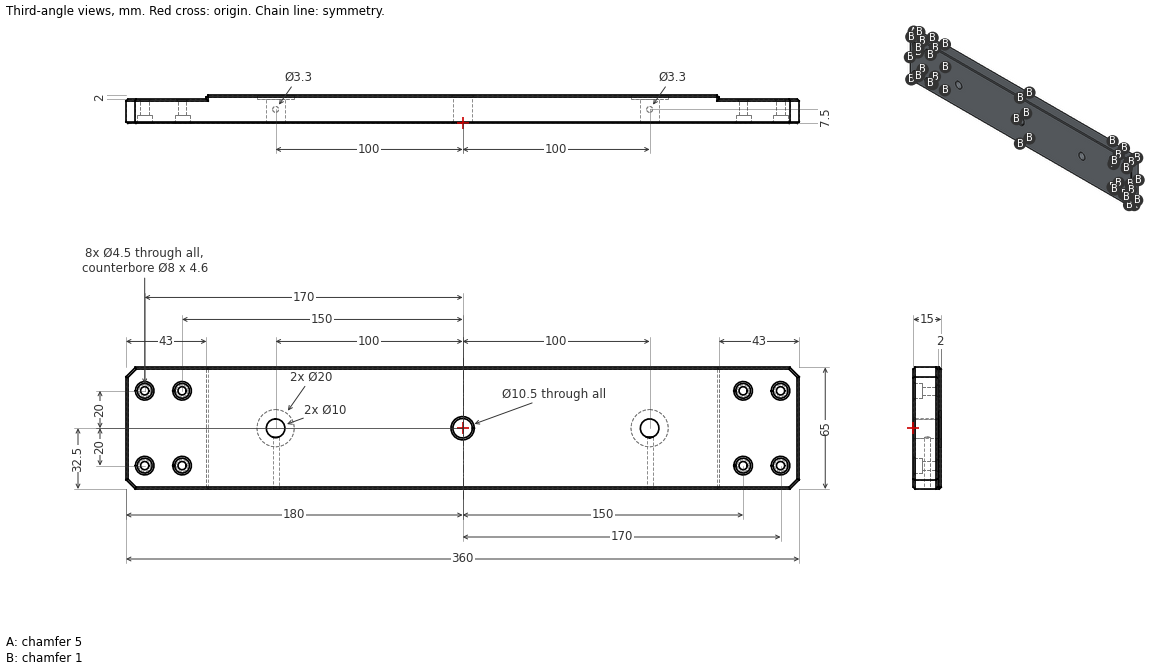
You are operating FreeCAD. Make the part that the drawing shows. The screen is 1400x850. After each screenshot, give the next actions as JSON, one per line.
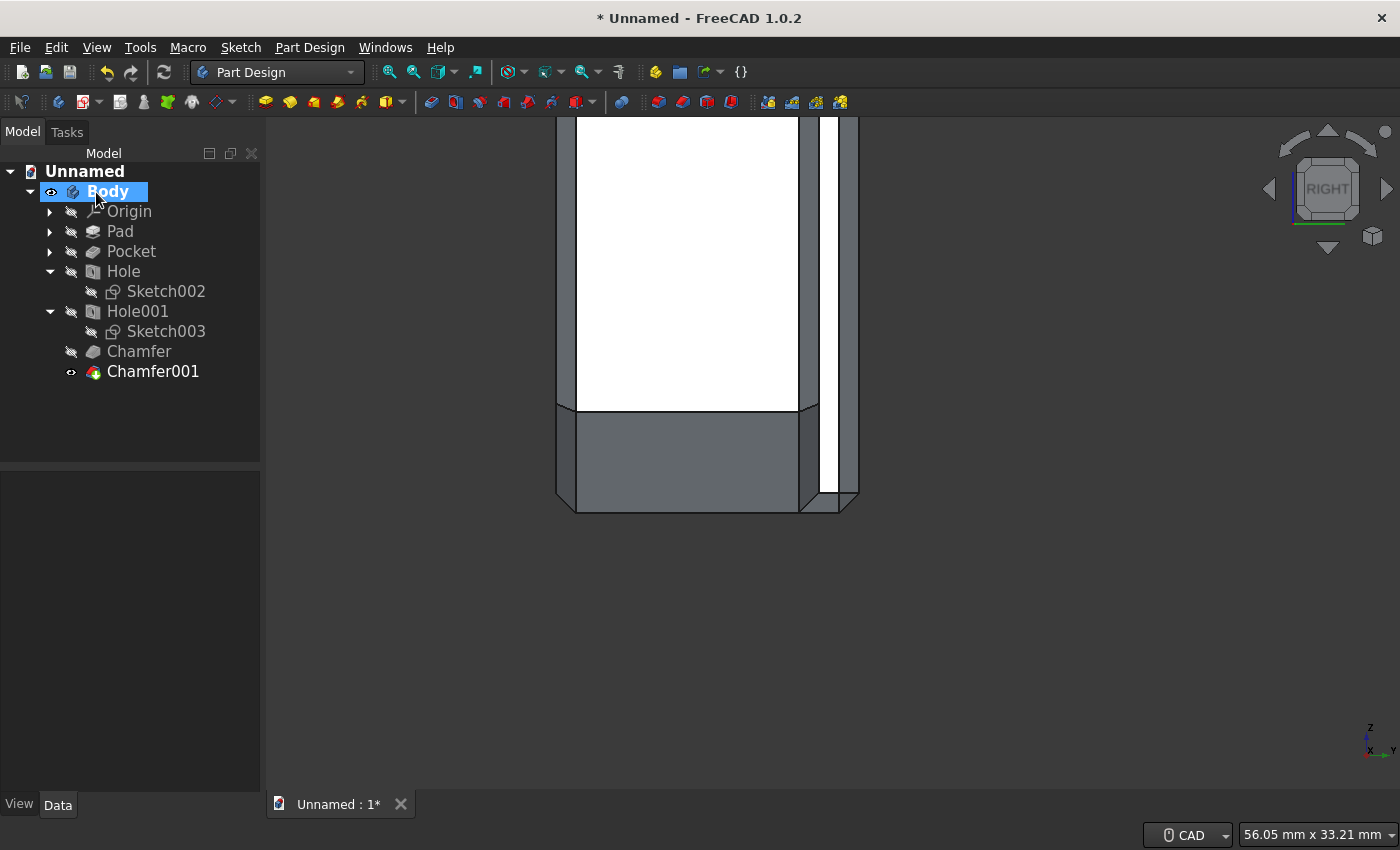
{"action": "left_click", "coordinate": [390, 72]}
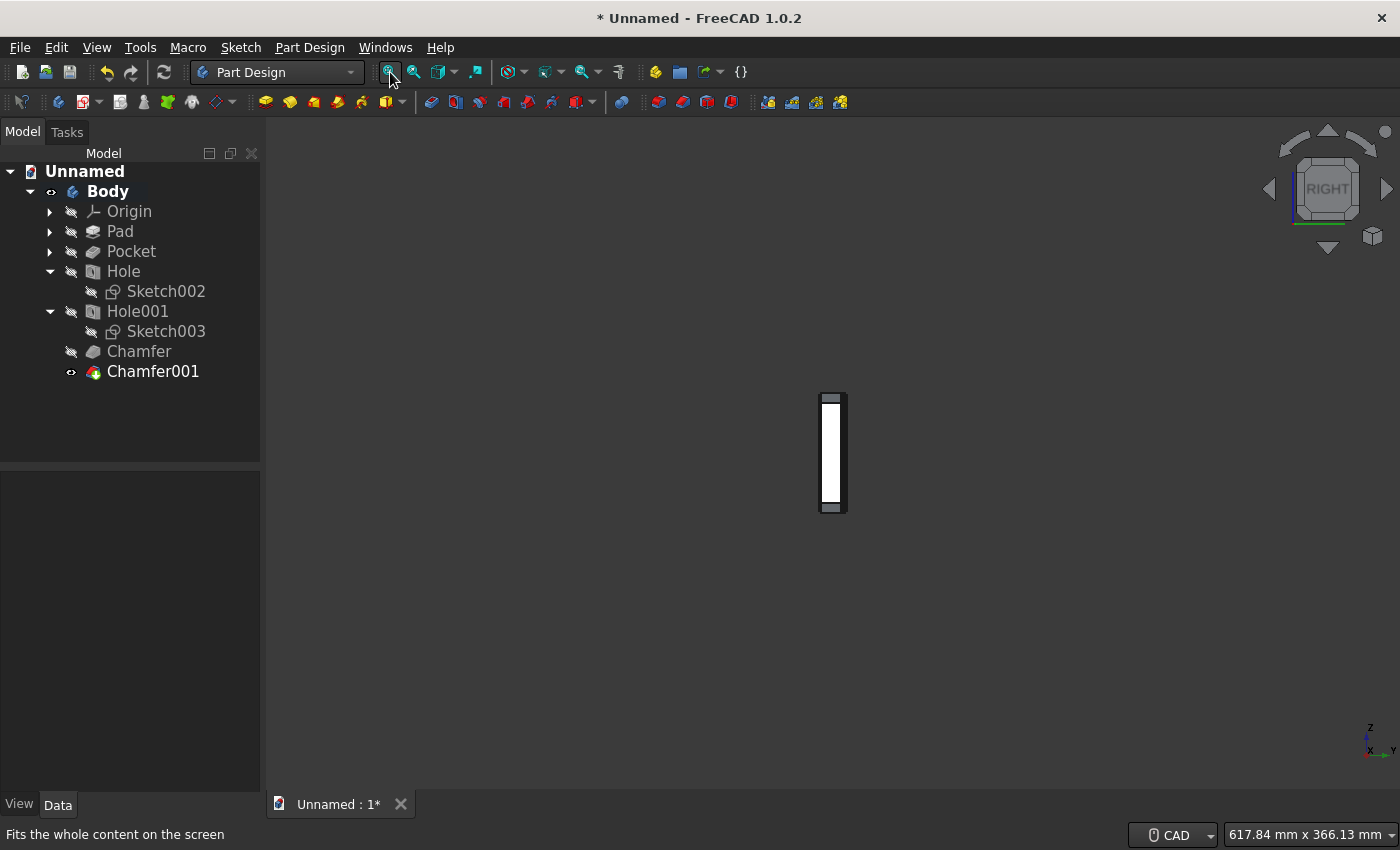
{"action": "key", "text": "4"}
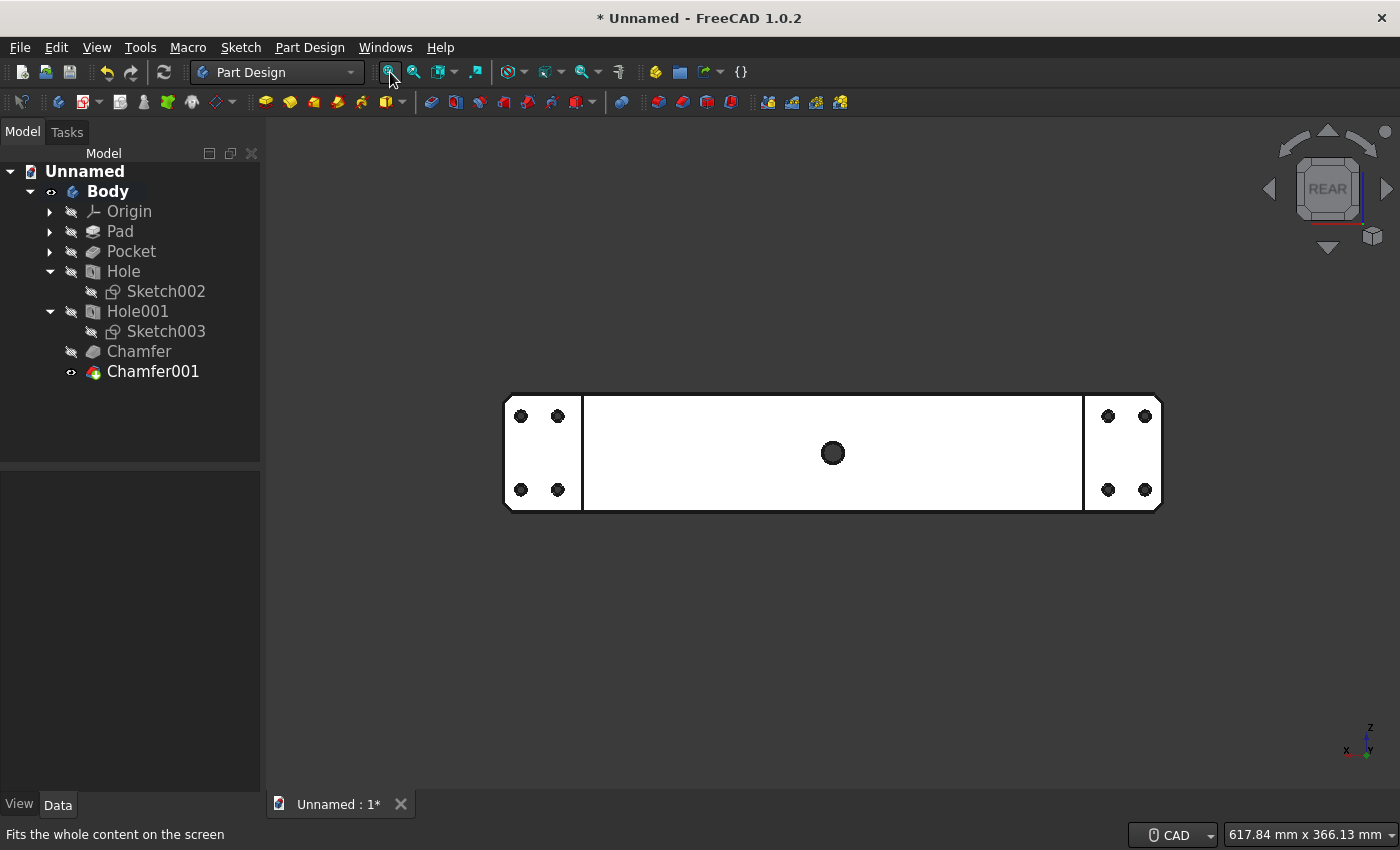
{"action": "left_click", "coordinate": [690, 452]}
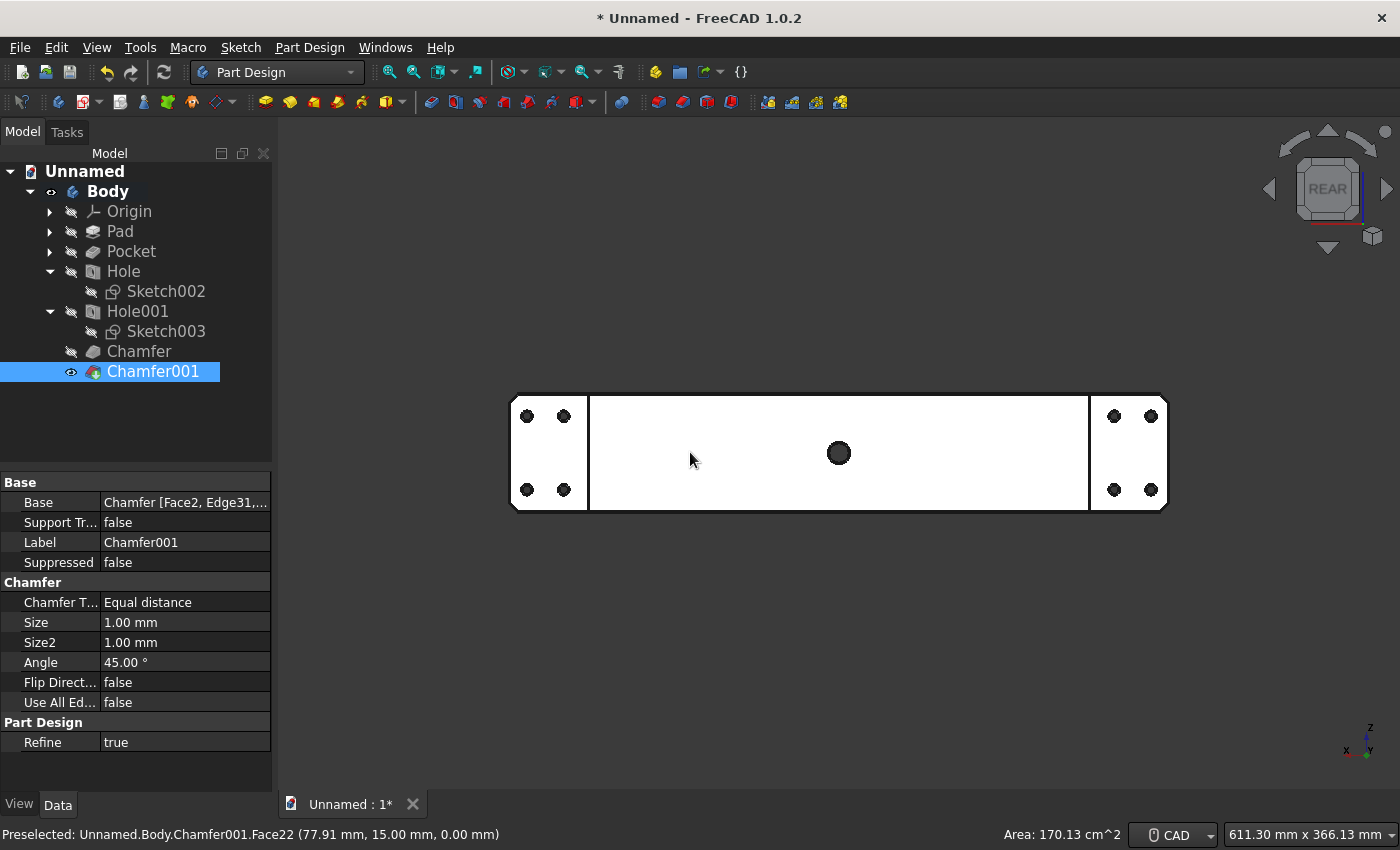
{"action": "left_click", "coordinate": [84, 102]}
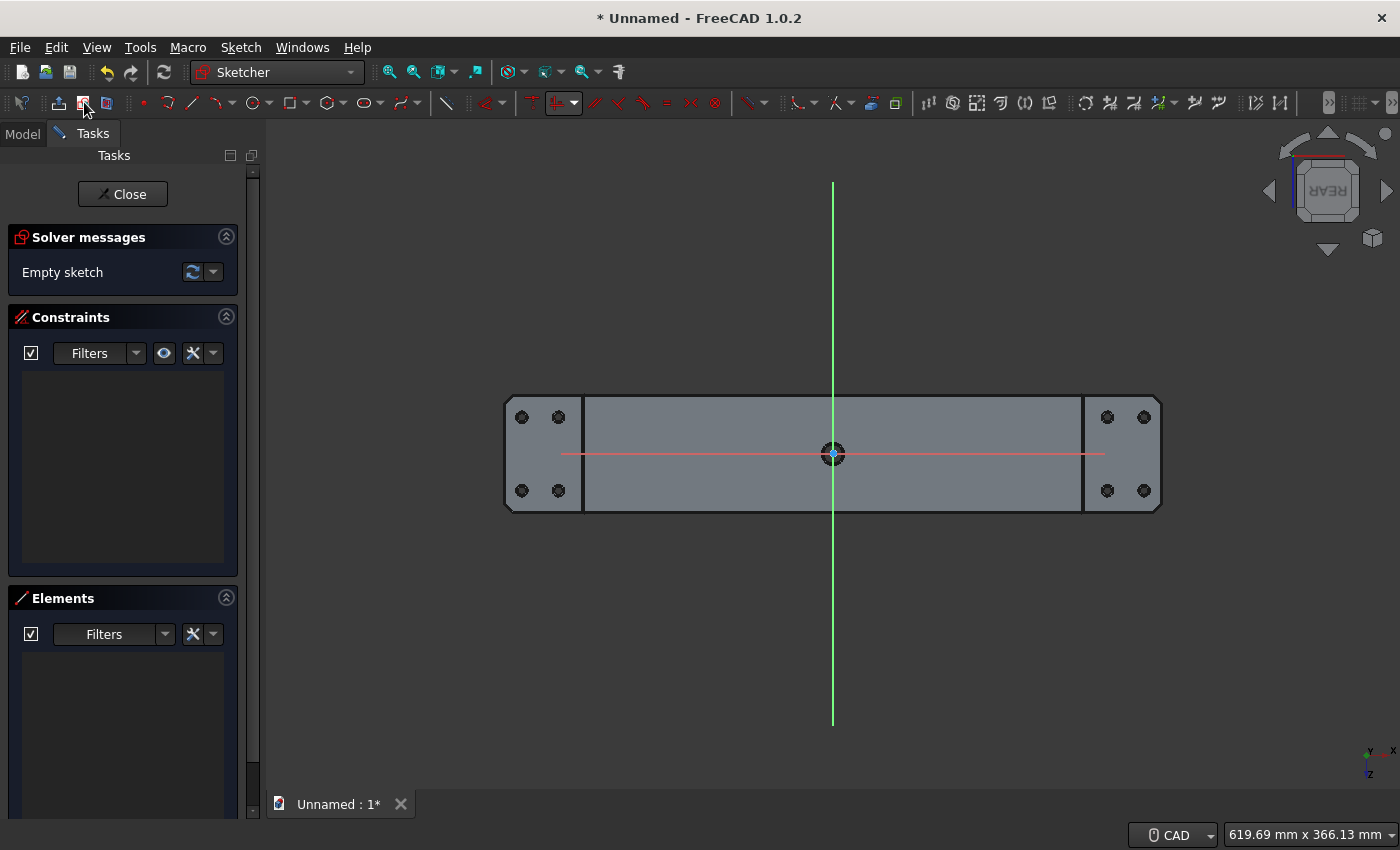
{"action": "scroll", "coordinate": [916, 454], "scroll_direction": "up", "scroll_amount": 3}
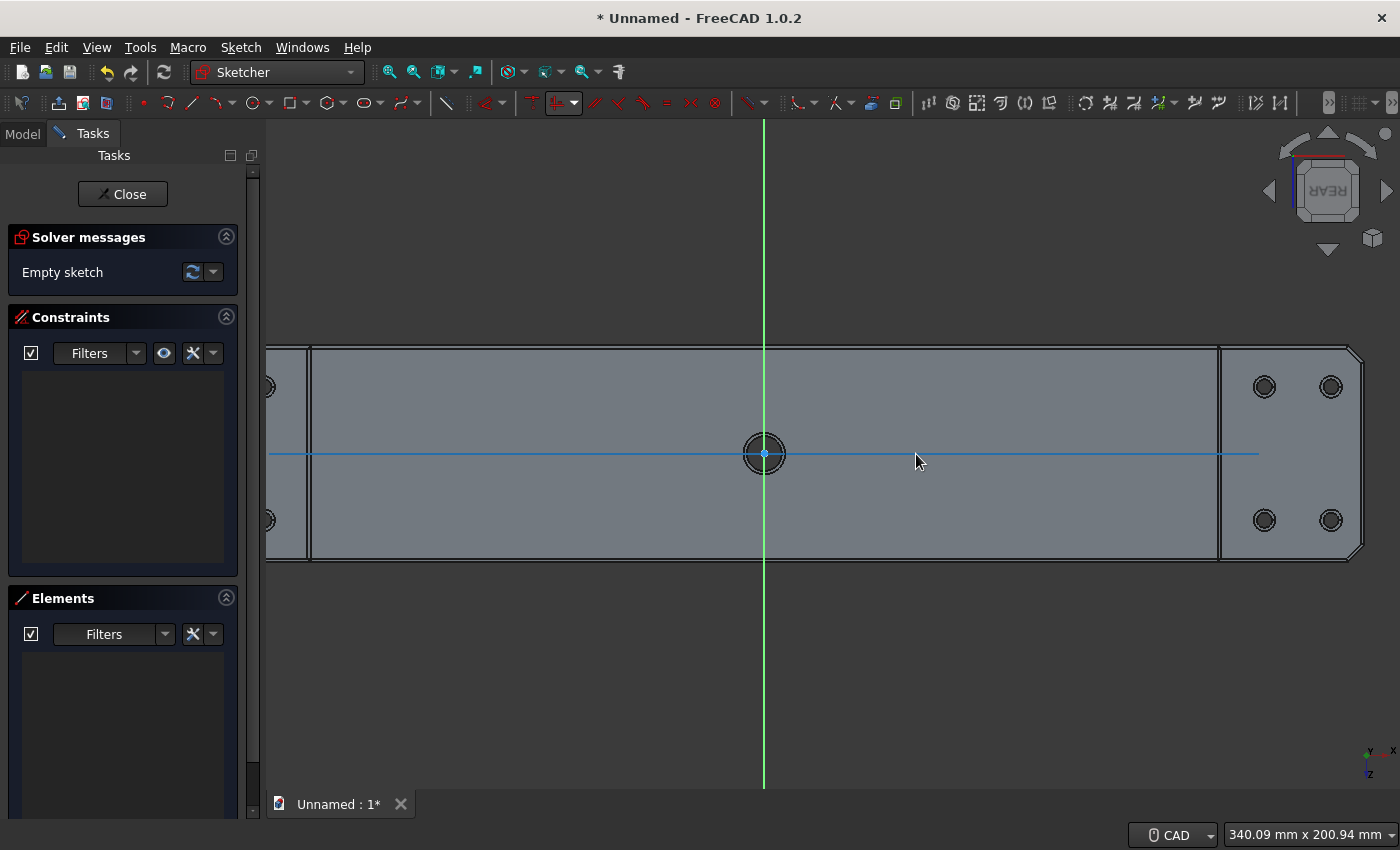
{"action": "left_click", "coordinate": [254, 104]}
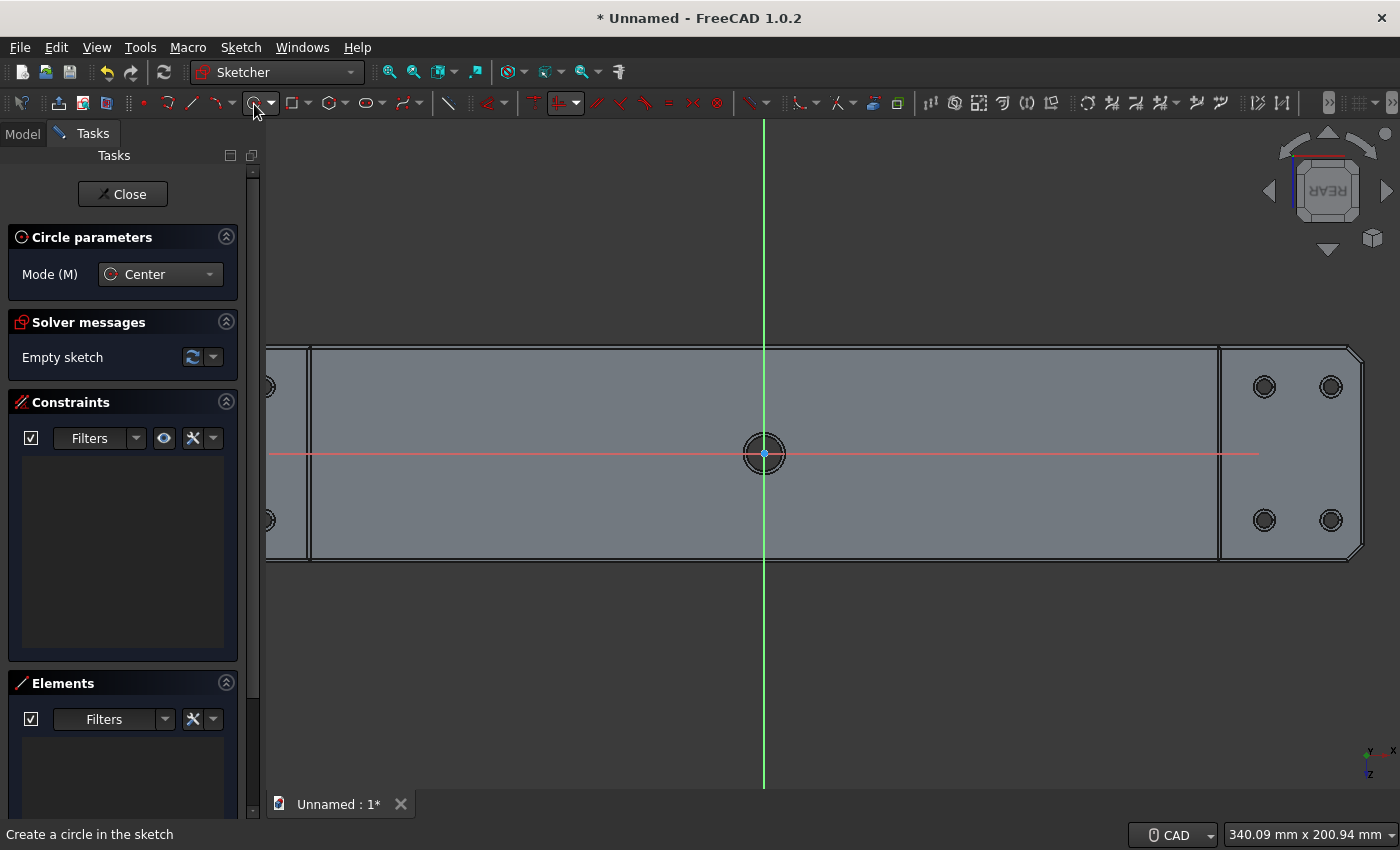
{"action": "scroll", "coordinate": [431, 454], "scroll_direction": "up", "scroll_amount": 2}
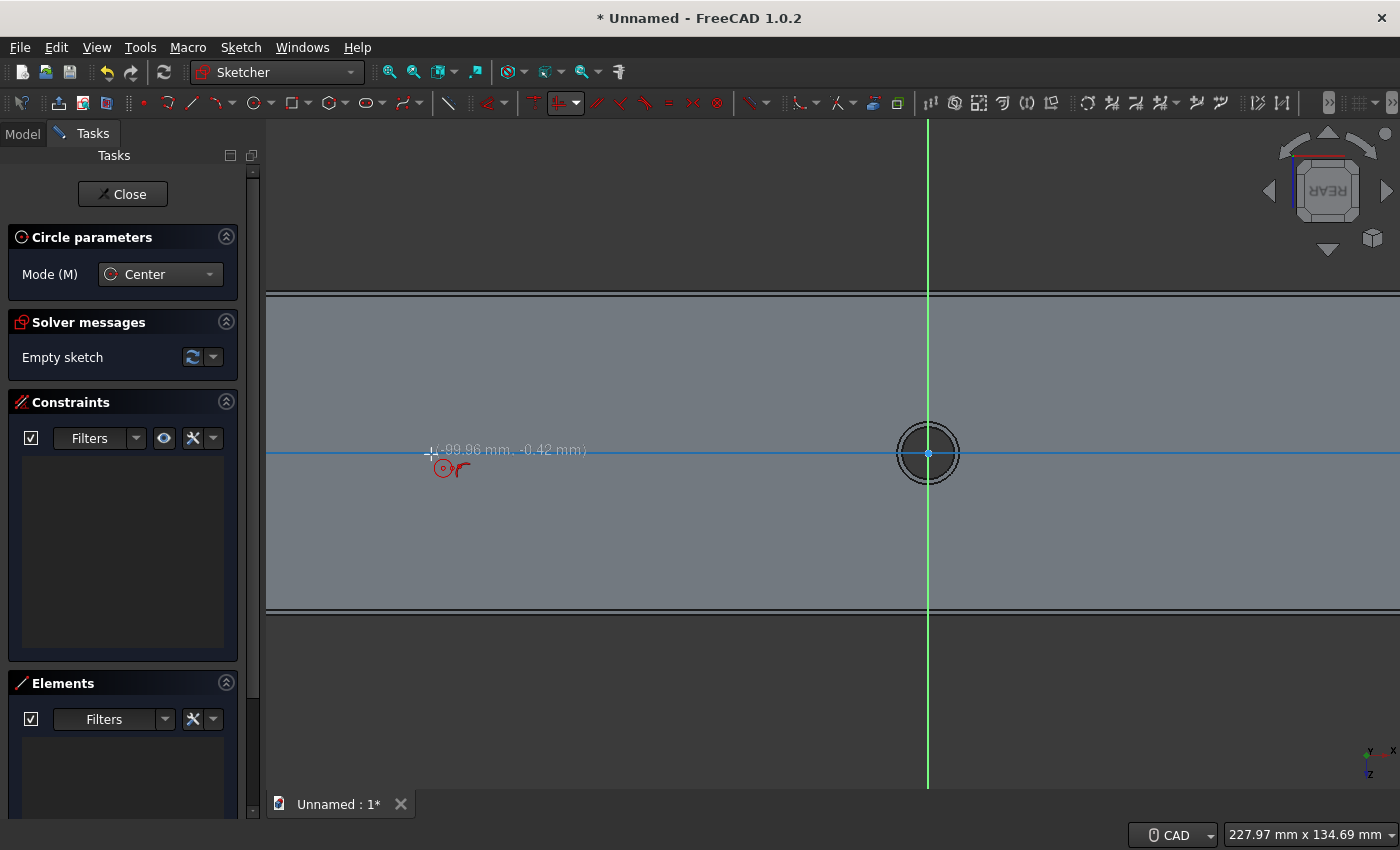
{"action": "left_click", "coordinate": [431, 453]}
{"action": "mouse_move", "coordinate": [448, 436]}